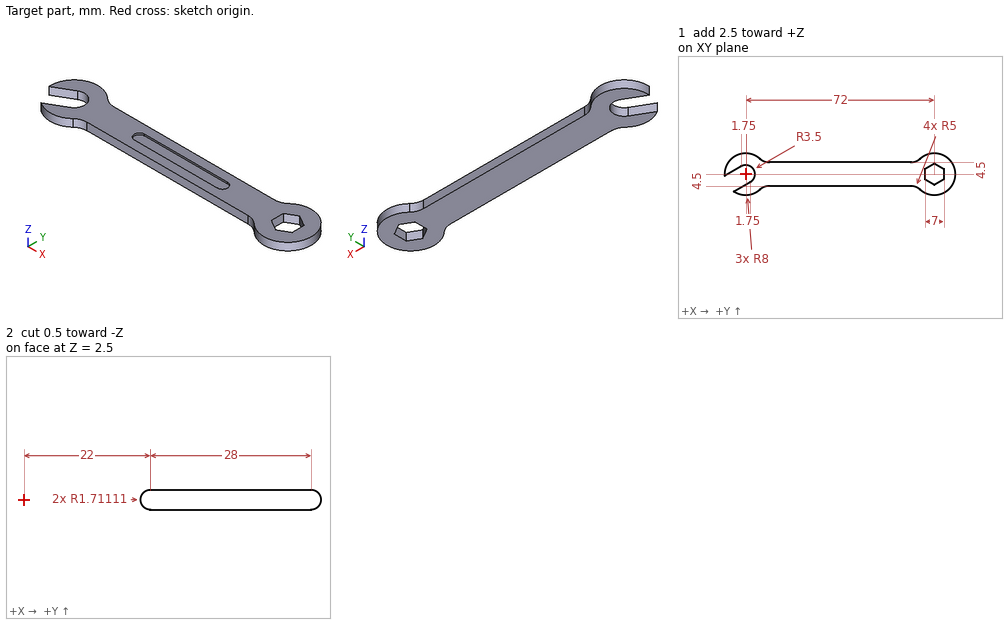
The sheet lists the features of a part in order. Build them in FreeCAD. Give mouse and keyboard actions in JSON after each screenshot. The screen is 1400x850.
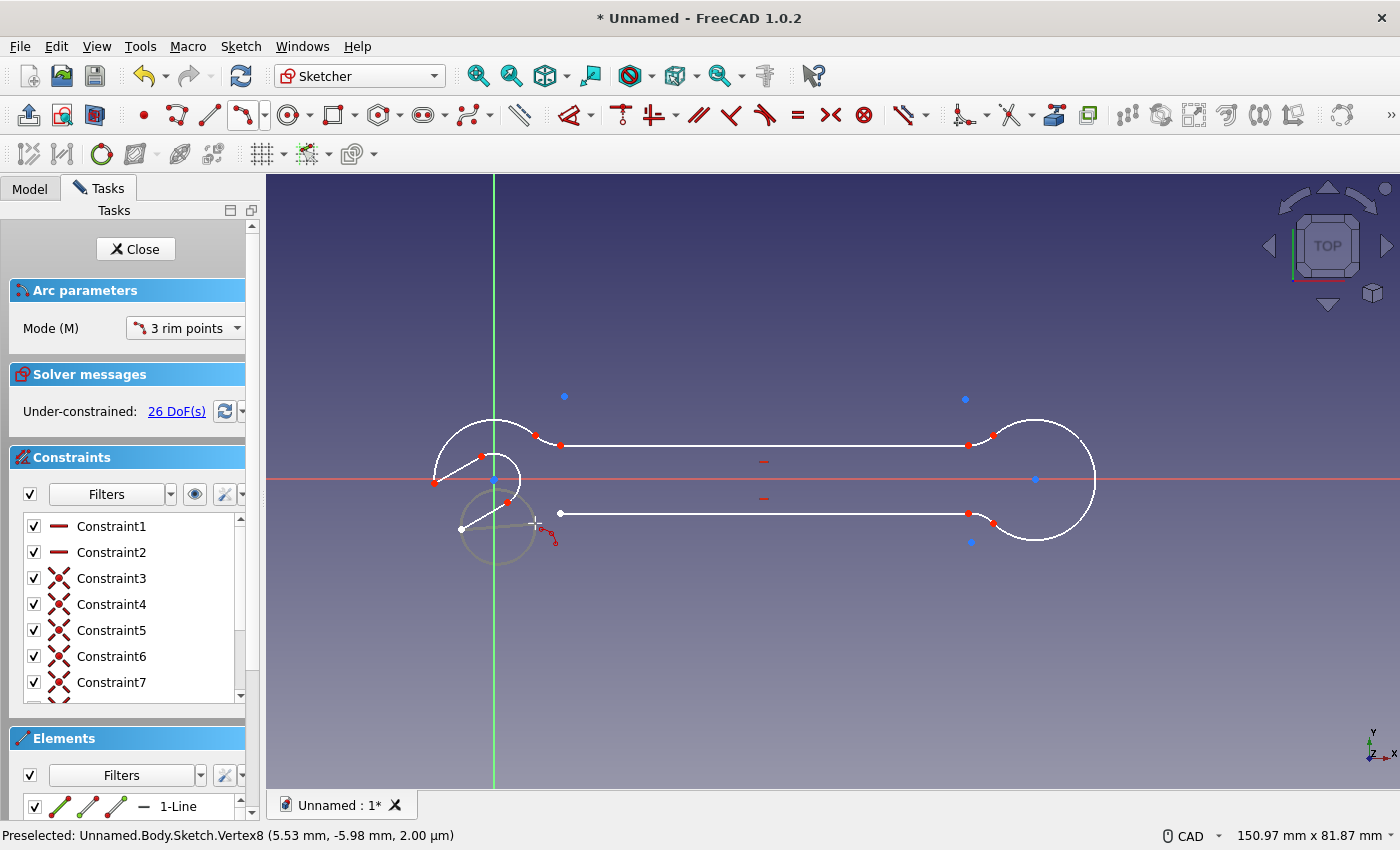
{"action": "scroll", "coordinate": [507, 538], "scroll_direction": "up", "scroll_amount": 2}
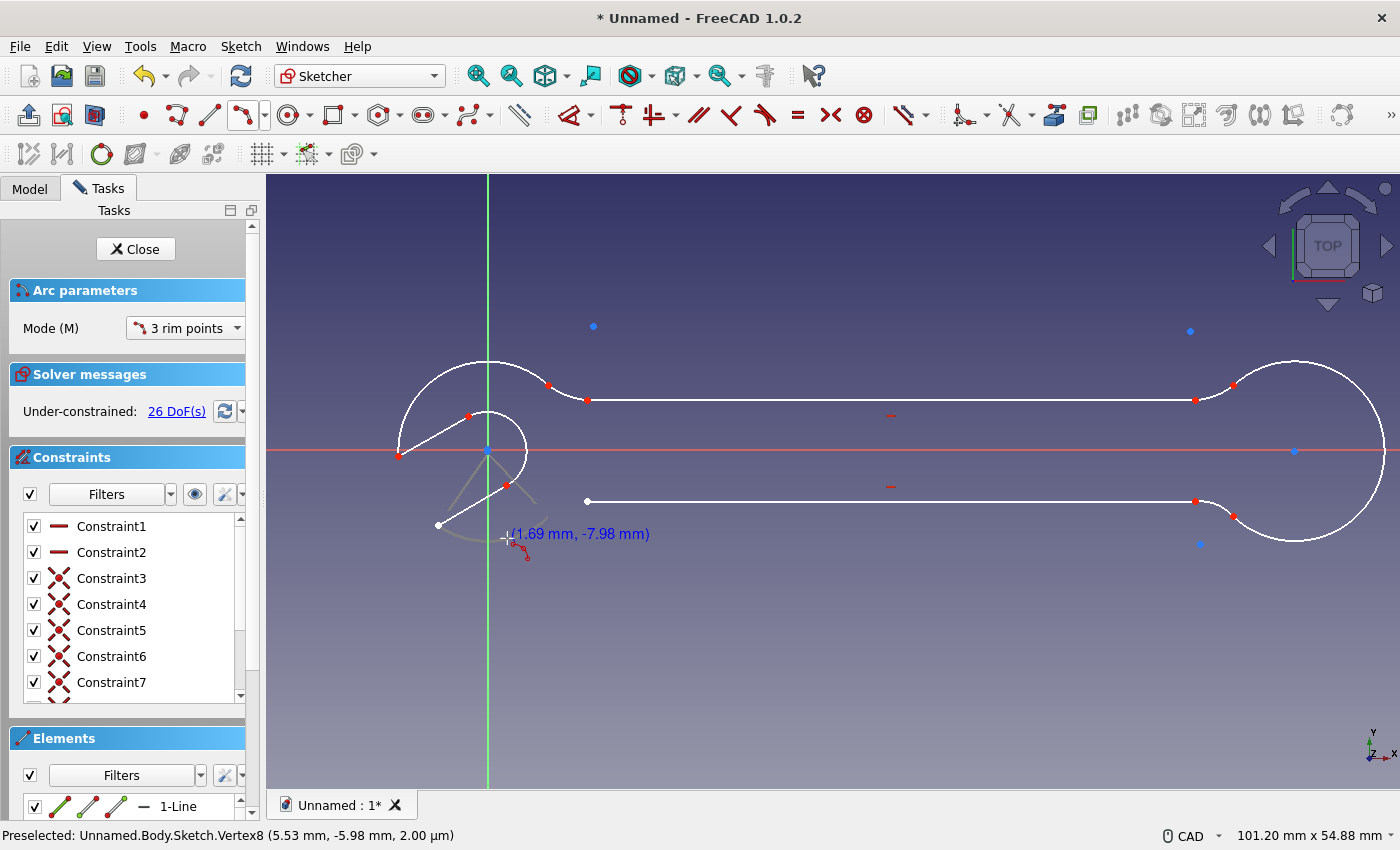
{"action": "left_click", "coordinate": [507, 537]}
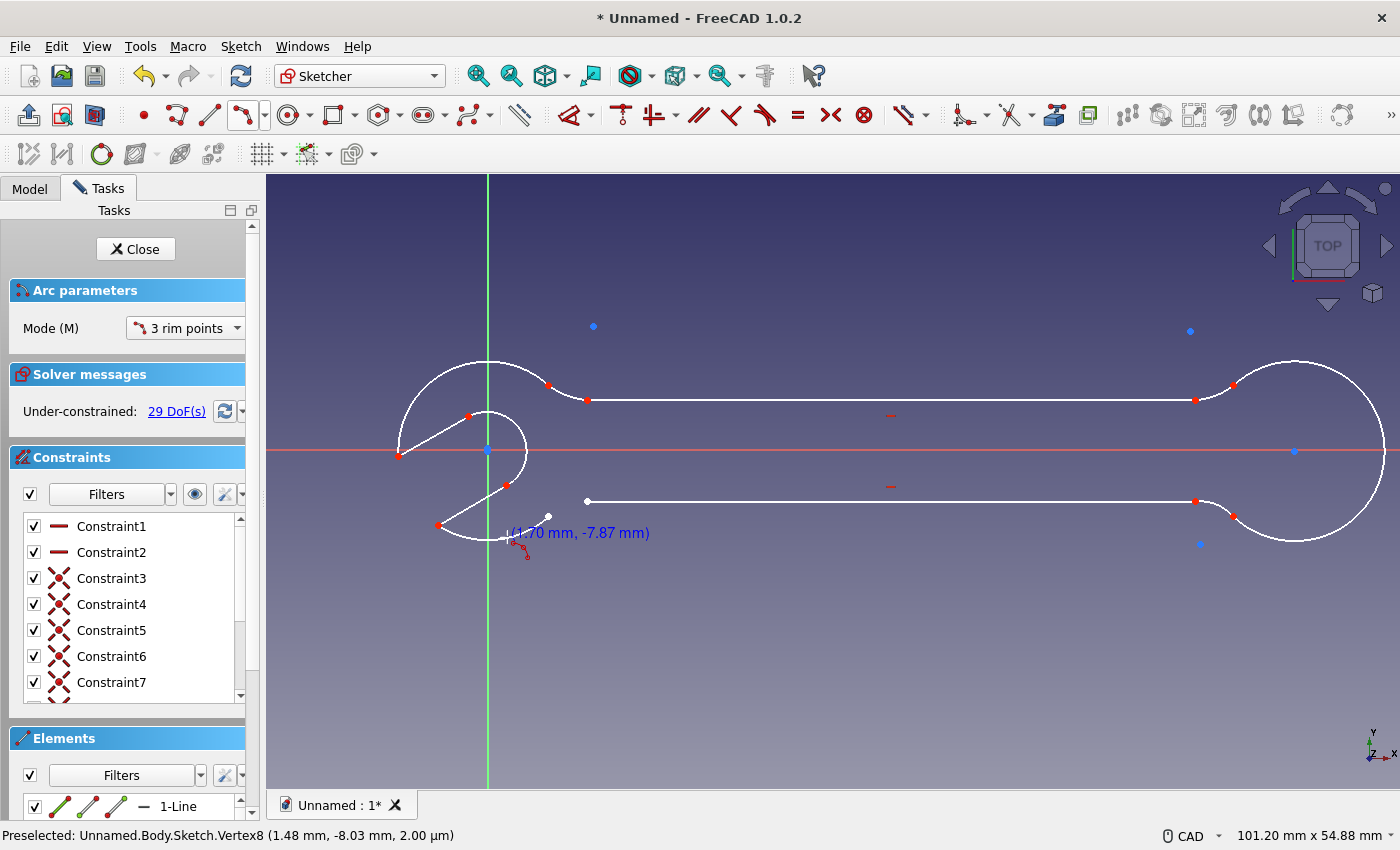
{"action": "left_click", "coordinate": [549, 517]}
{"action": "left_click", "coordinate": [587, 502]}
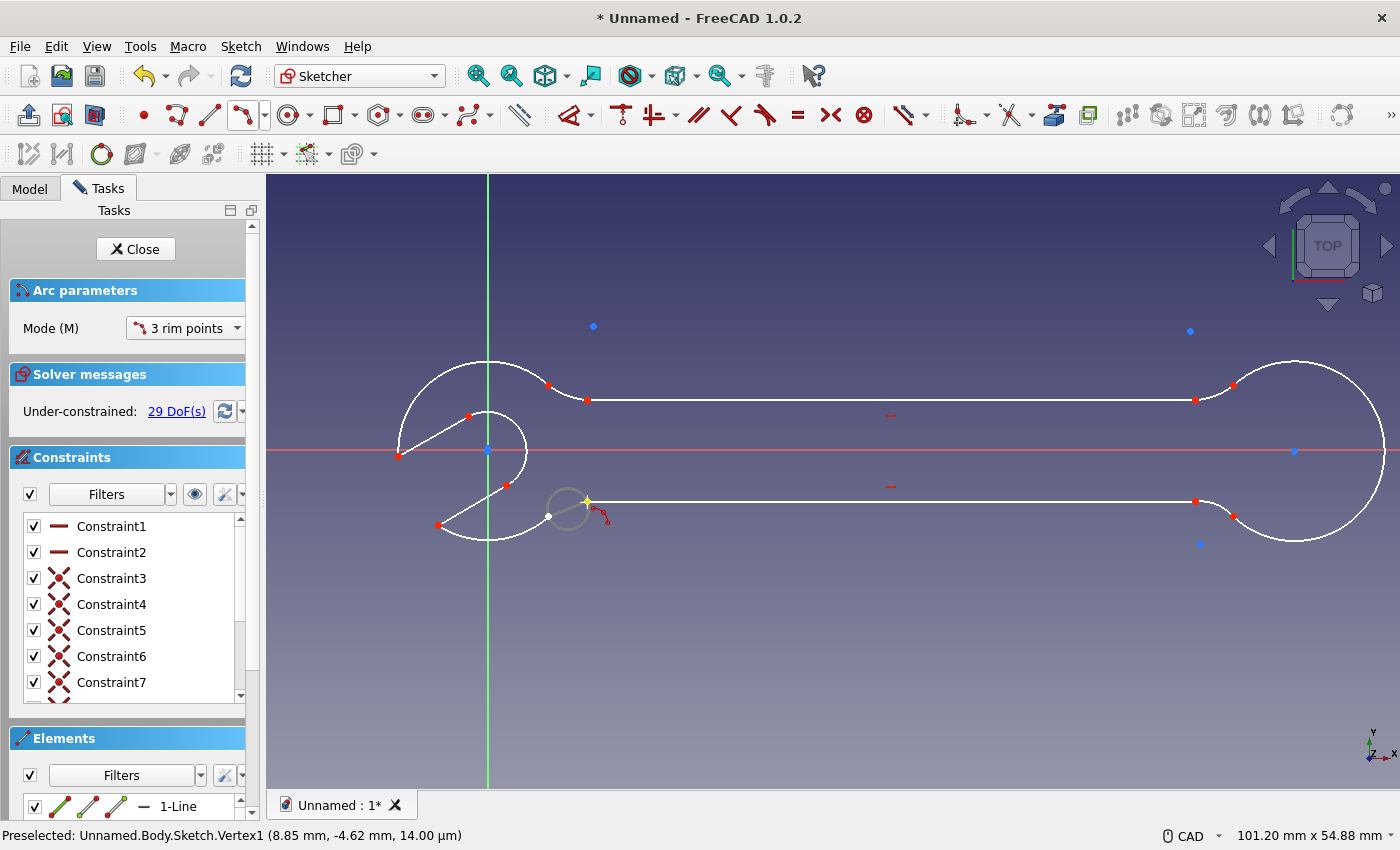
{"action": "scroll", "coordinate": [567, 504], "scroll_direction": "up", "scroll_amount": 8}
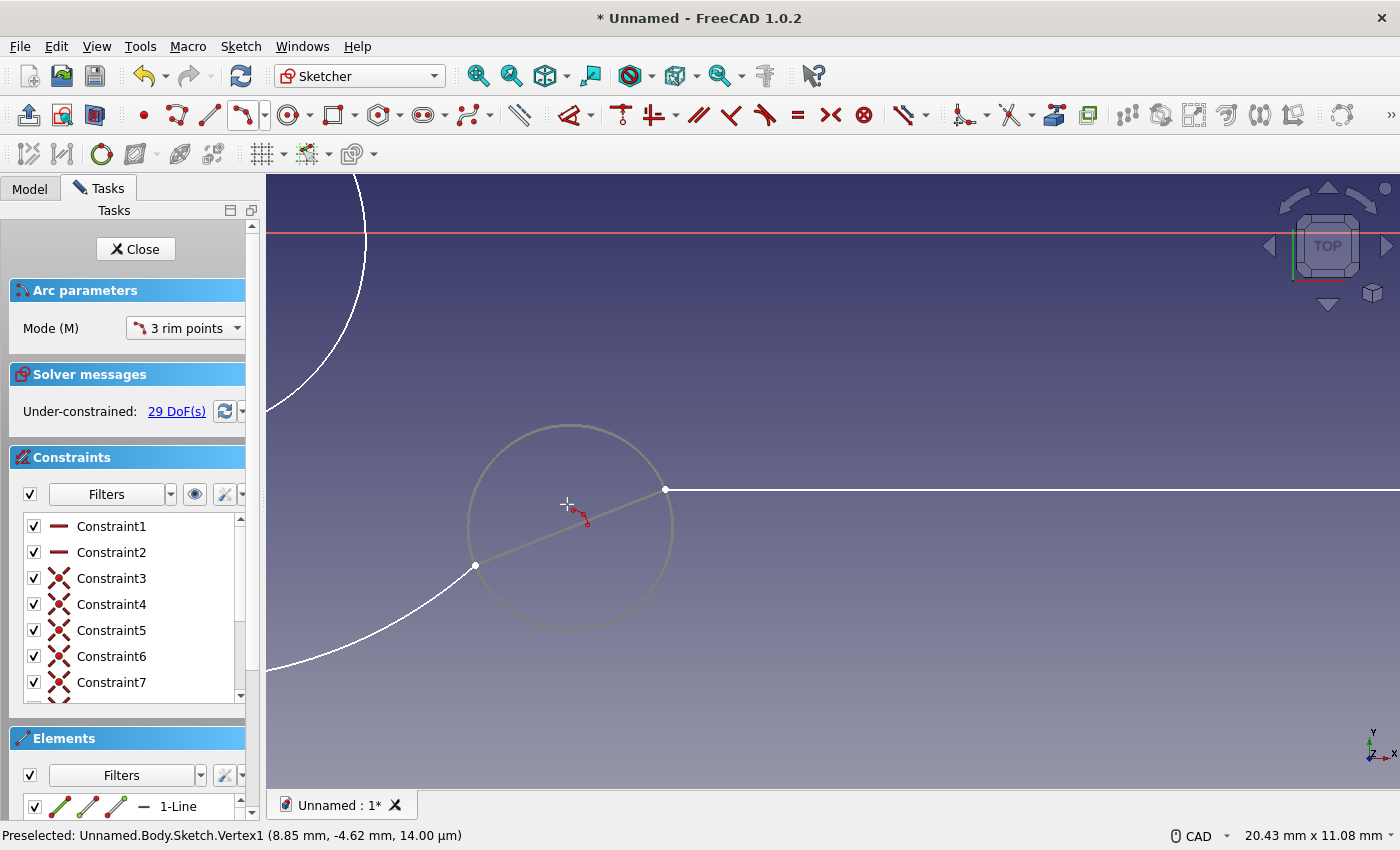
{"action": "left_click", "coordinate": [565, 502]}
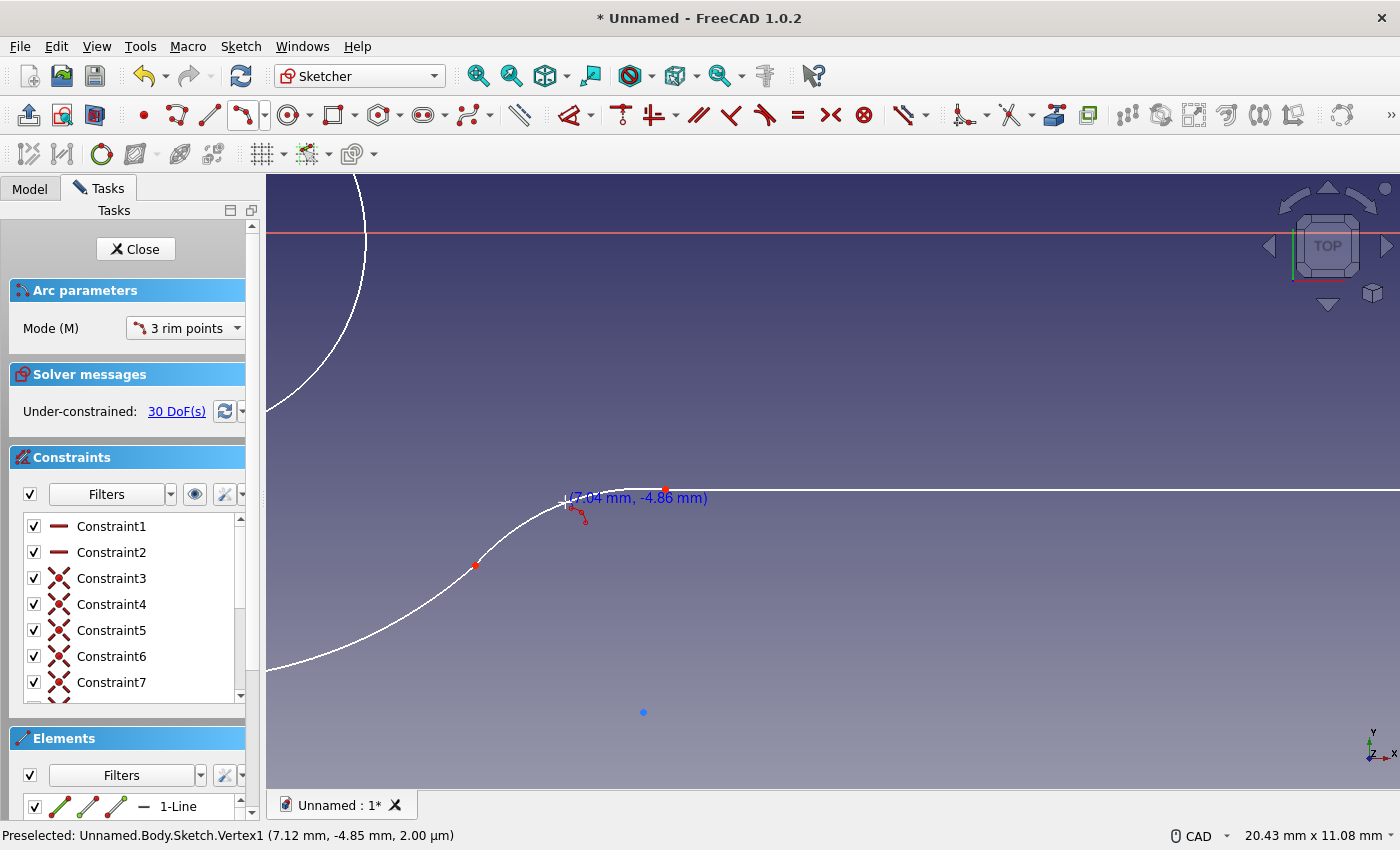
{"action": "key", "text": "g p 6"}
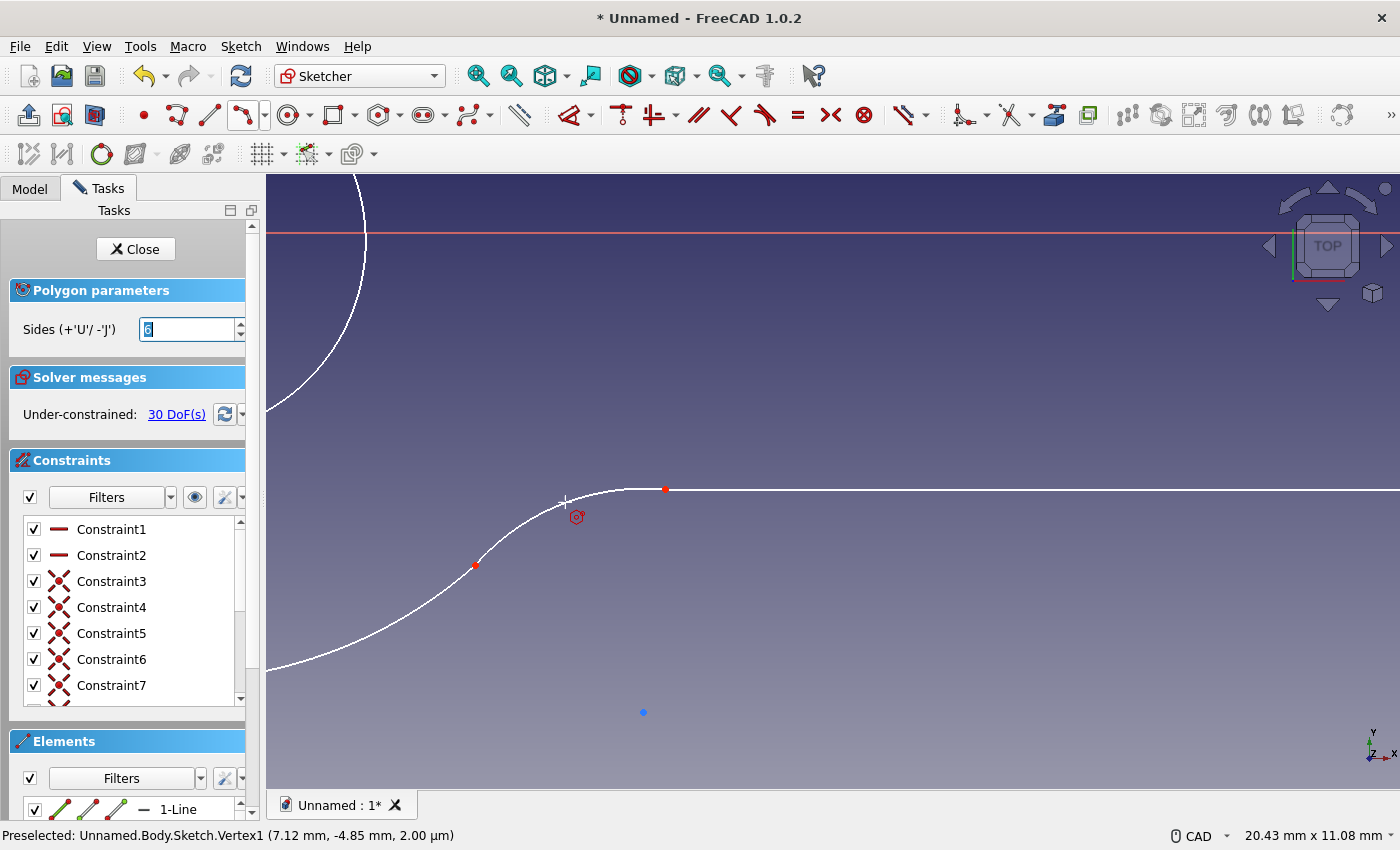
{"action": "scroll", "coordinate": [544, 517], "scroll_direction": "down", "scroll_amount": 10}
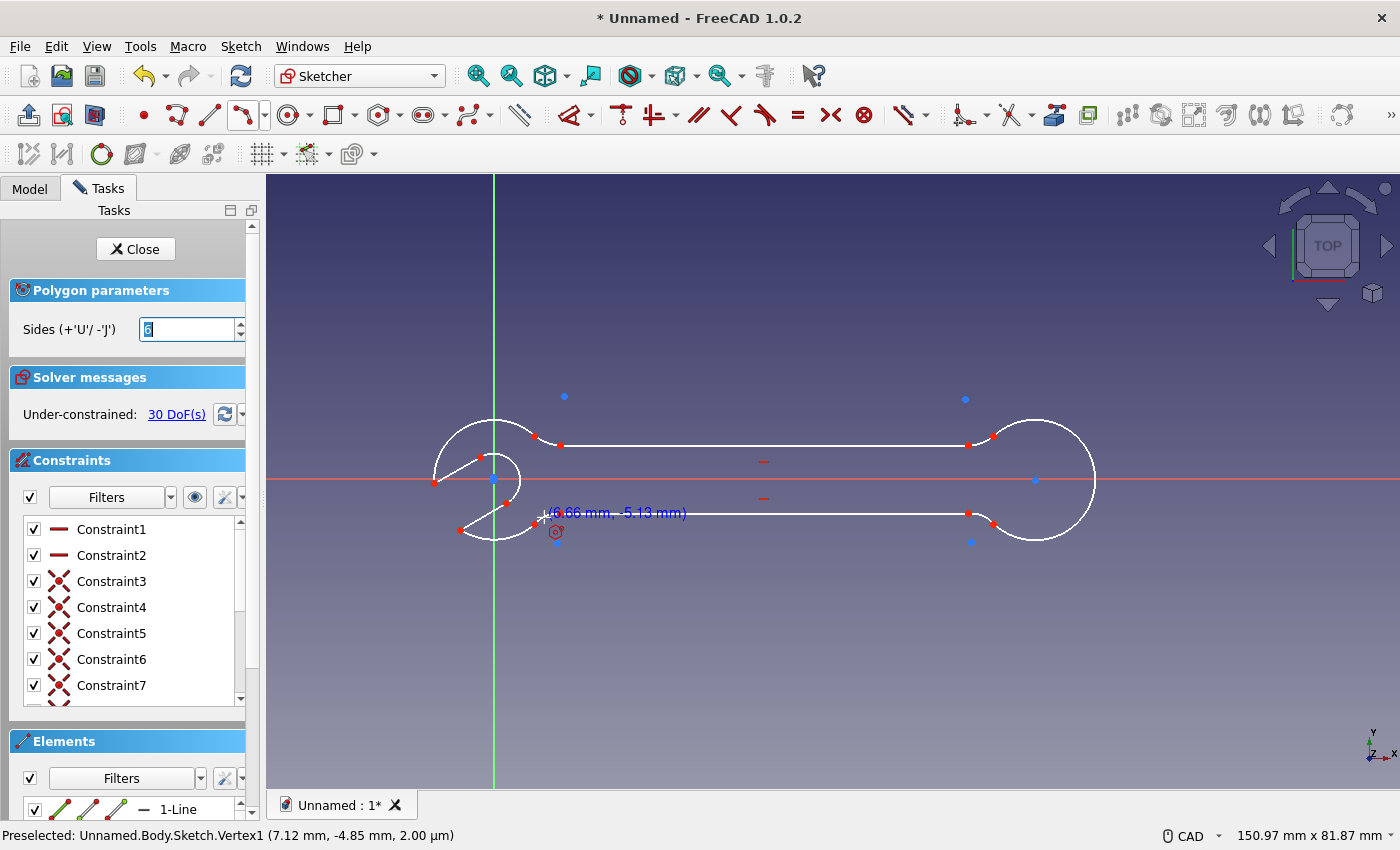
{"action": "left_click", "coordinate": [1035, 479]}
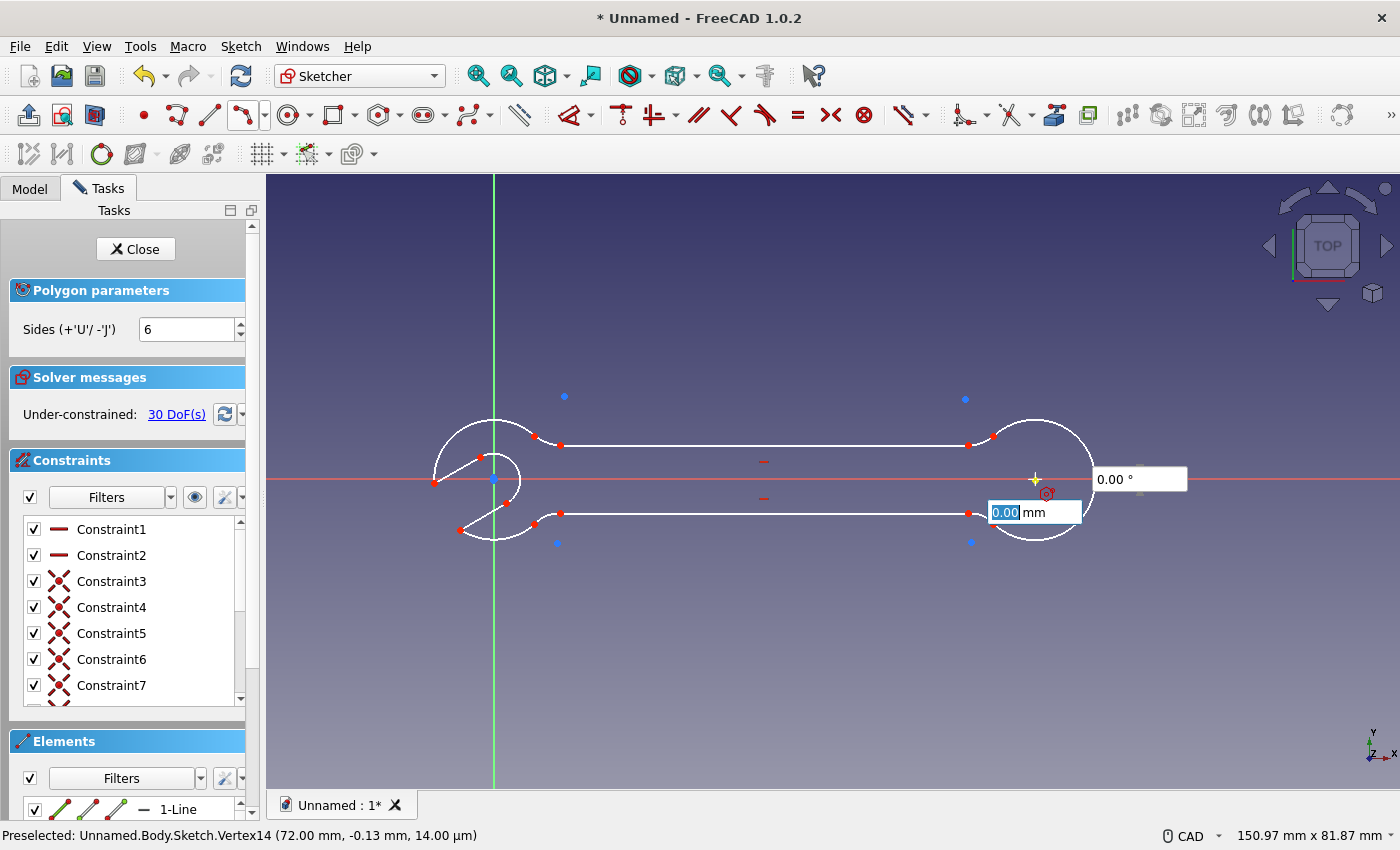
{"action": "left_click", "coordinate": [1035, 509]}
{"action": "key", "text": "Escape"}